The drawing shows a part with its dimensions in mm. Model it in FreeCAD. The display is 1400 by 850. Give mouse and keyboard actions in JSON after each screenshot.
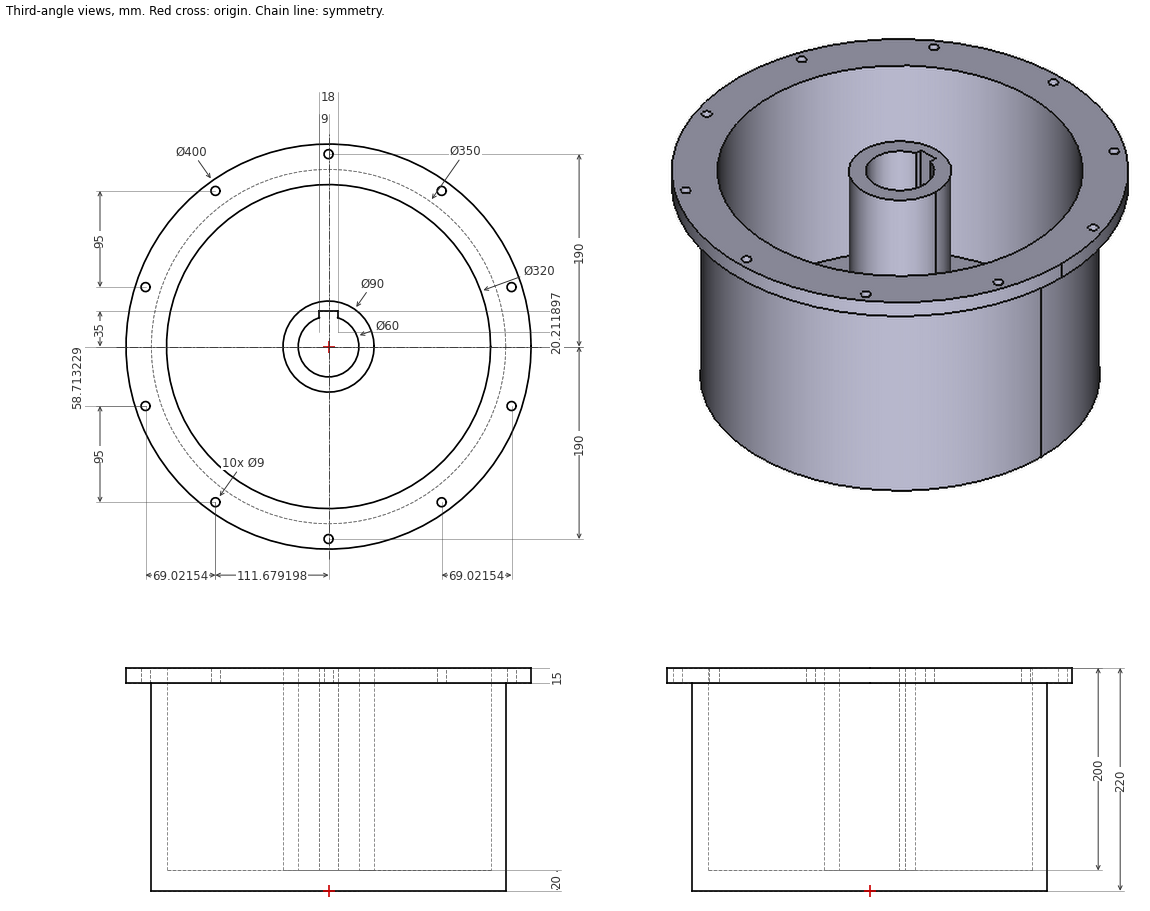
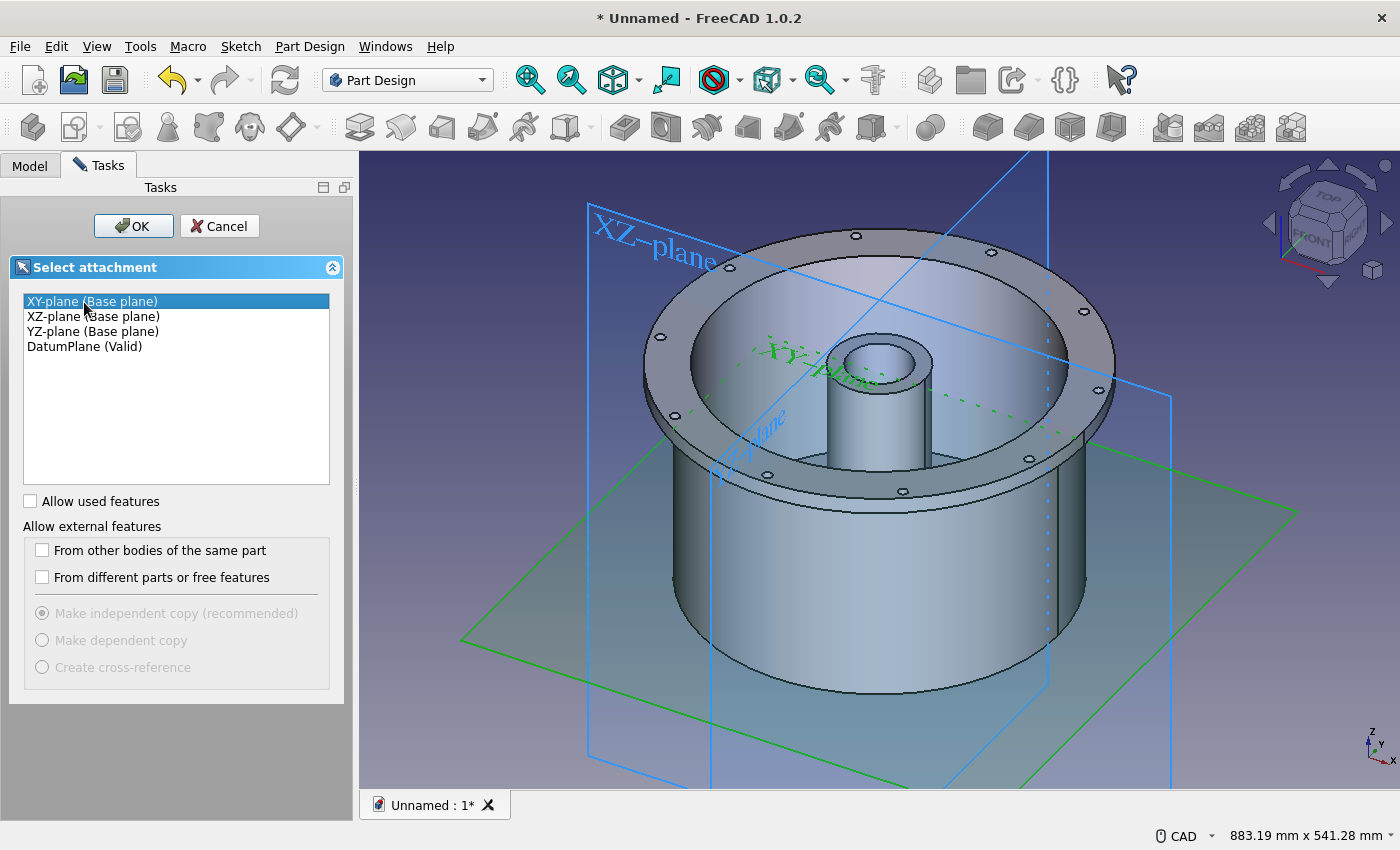
{"action": "left_click", "coordinate": [134, 226]}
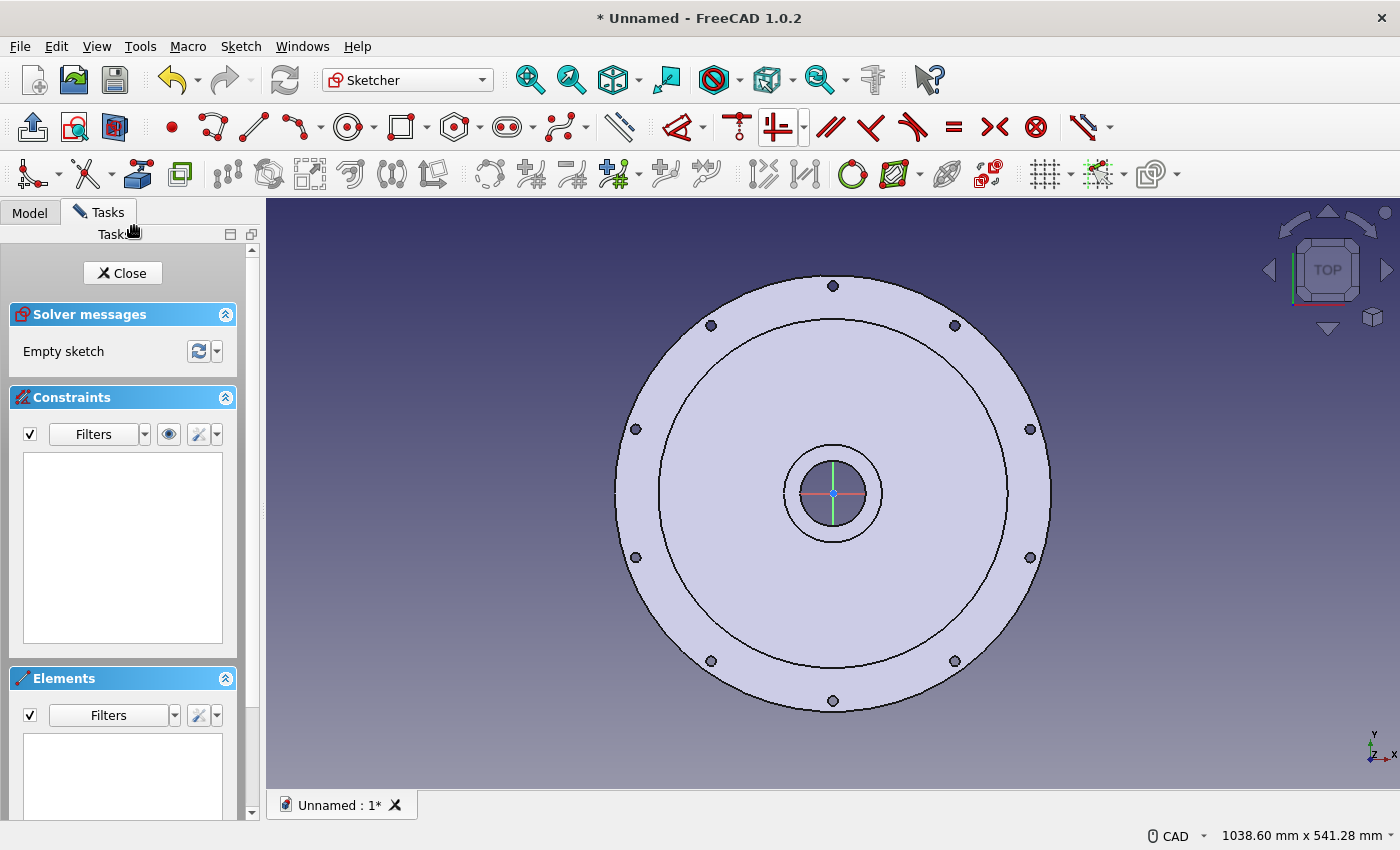
{"action": "left_click", "coordinate": [115, 128]}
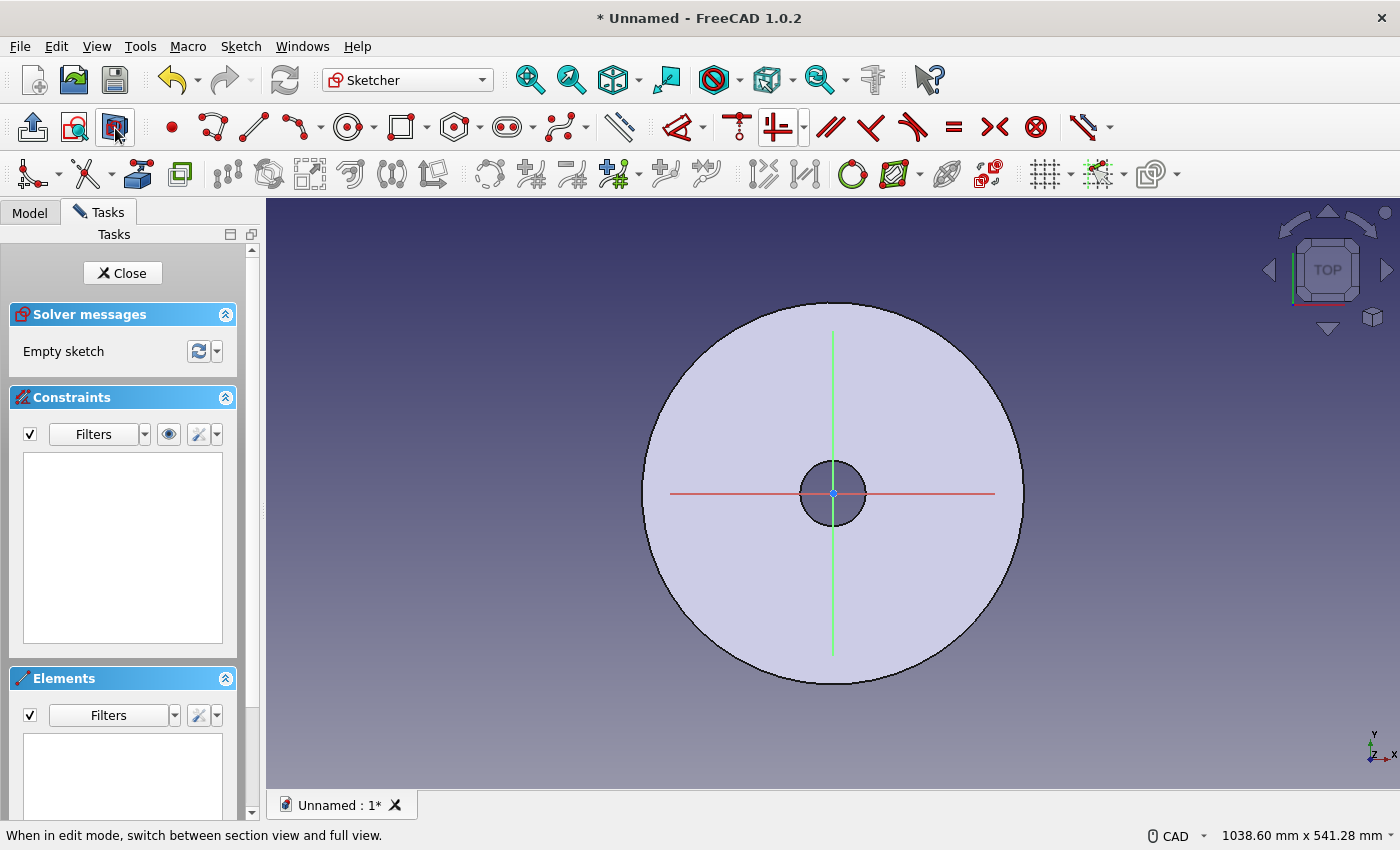
{"action": "scroll", "coordinate": [847, 494], "scroll_direction": "up", "scroll_amount": 9}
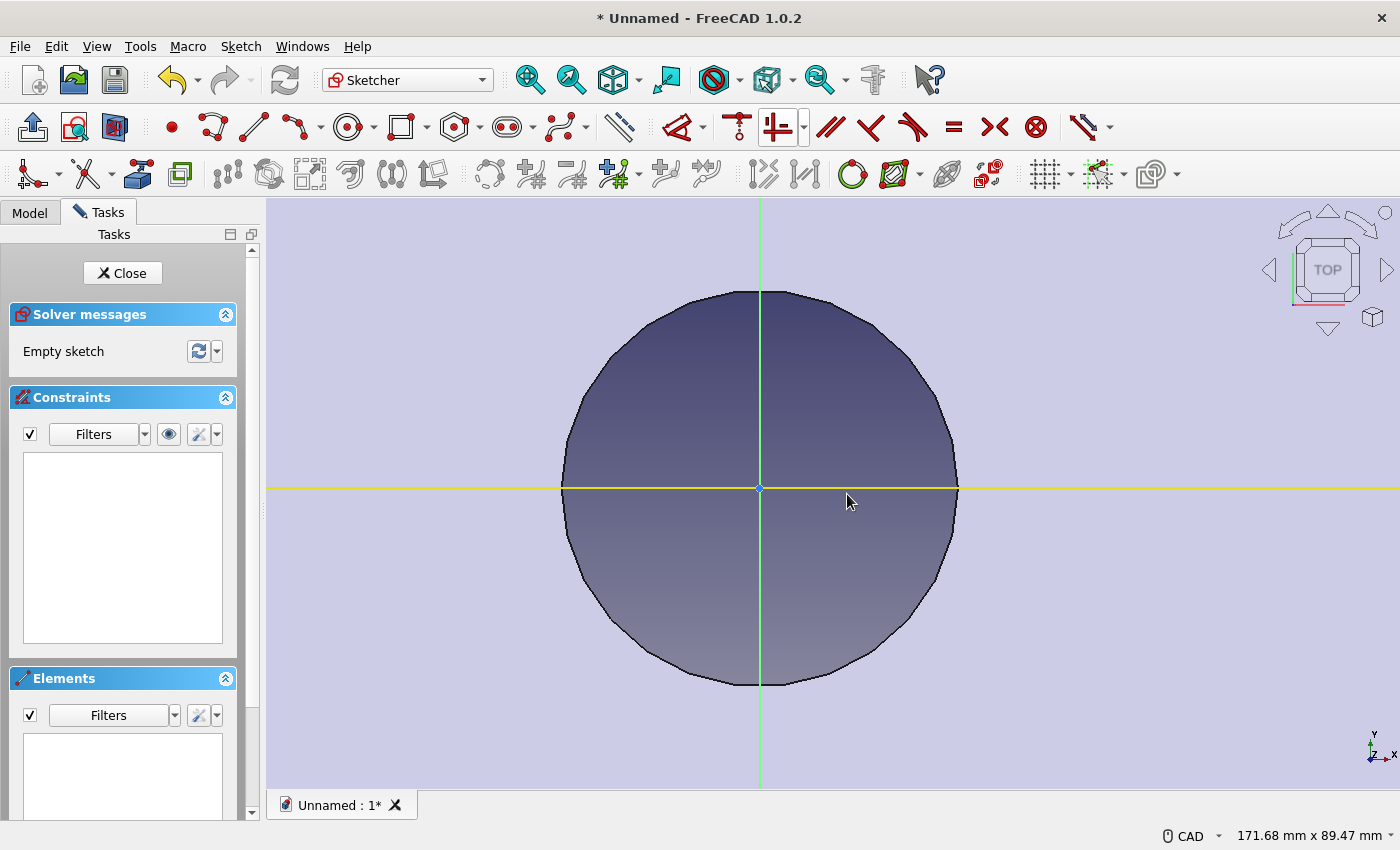
{"action": "left_click", "coordinate": [348, 128]}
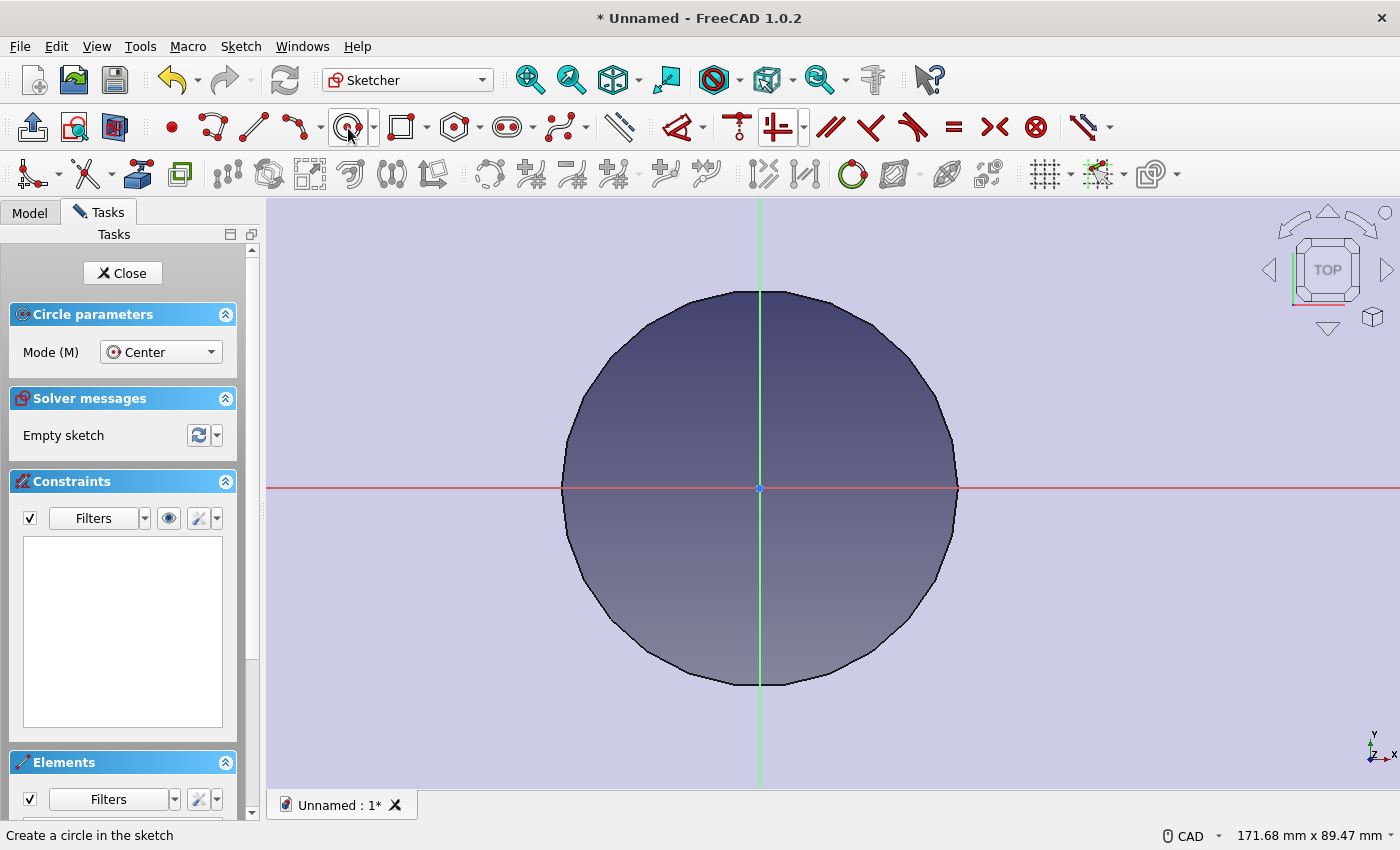
{"action": "left_click", "coordinate": [760, 488]}
{"action": "mouse_move", "coordinate": [900, 348]}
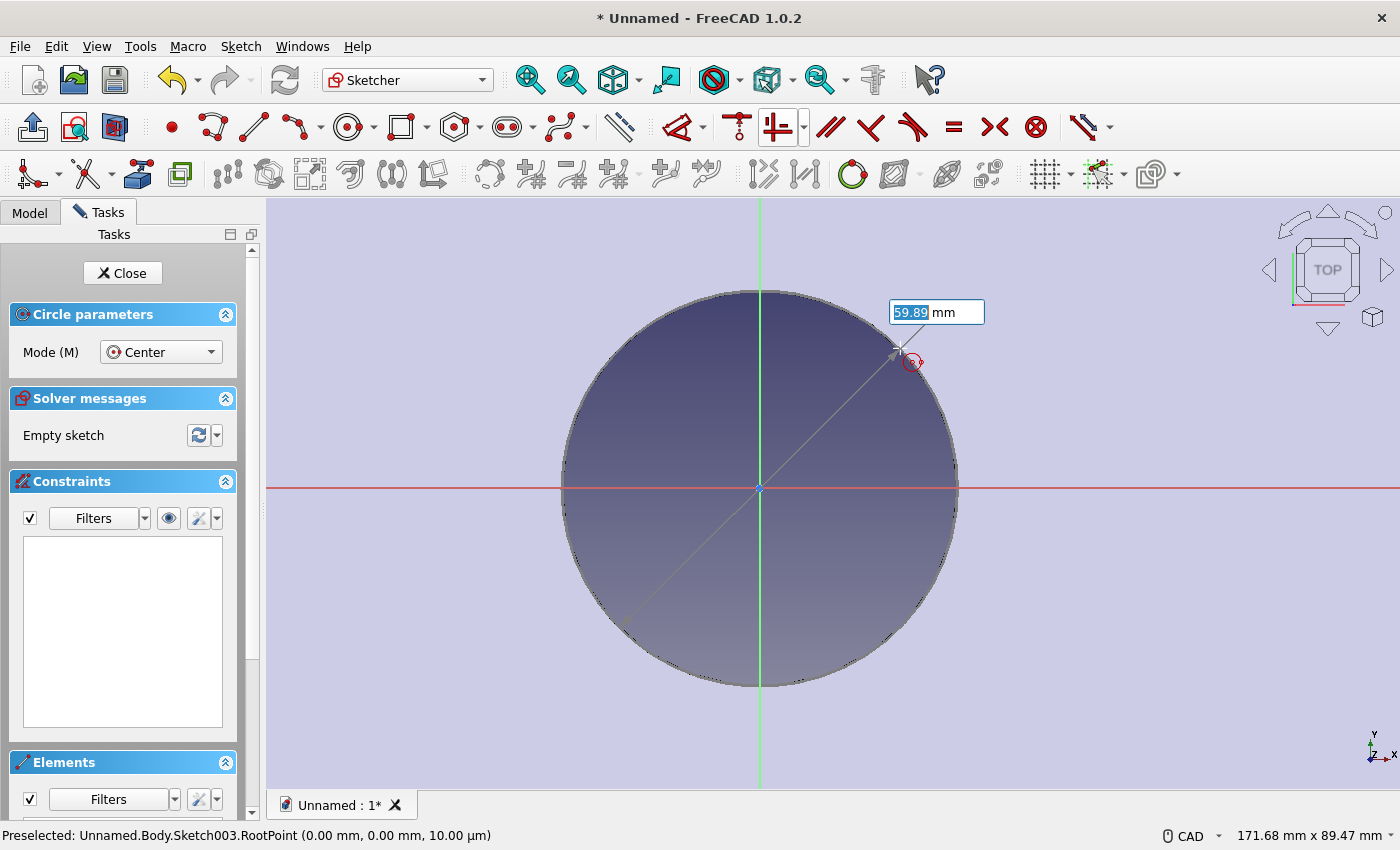
{"action": "type", "text": "60"}
{"action": "key", "text": "Return"}
{"action": "key", "text": "Escape"}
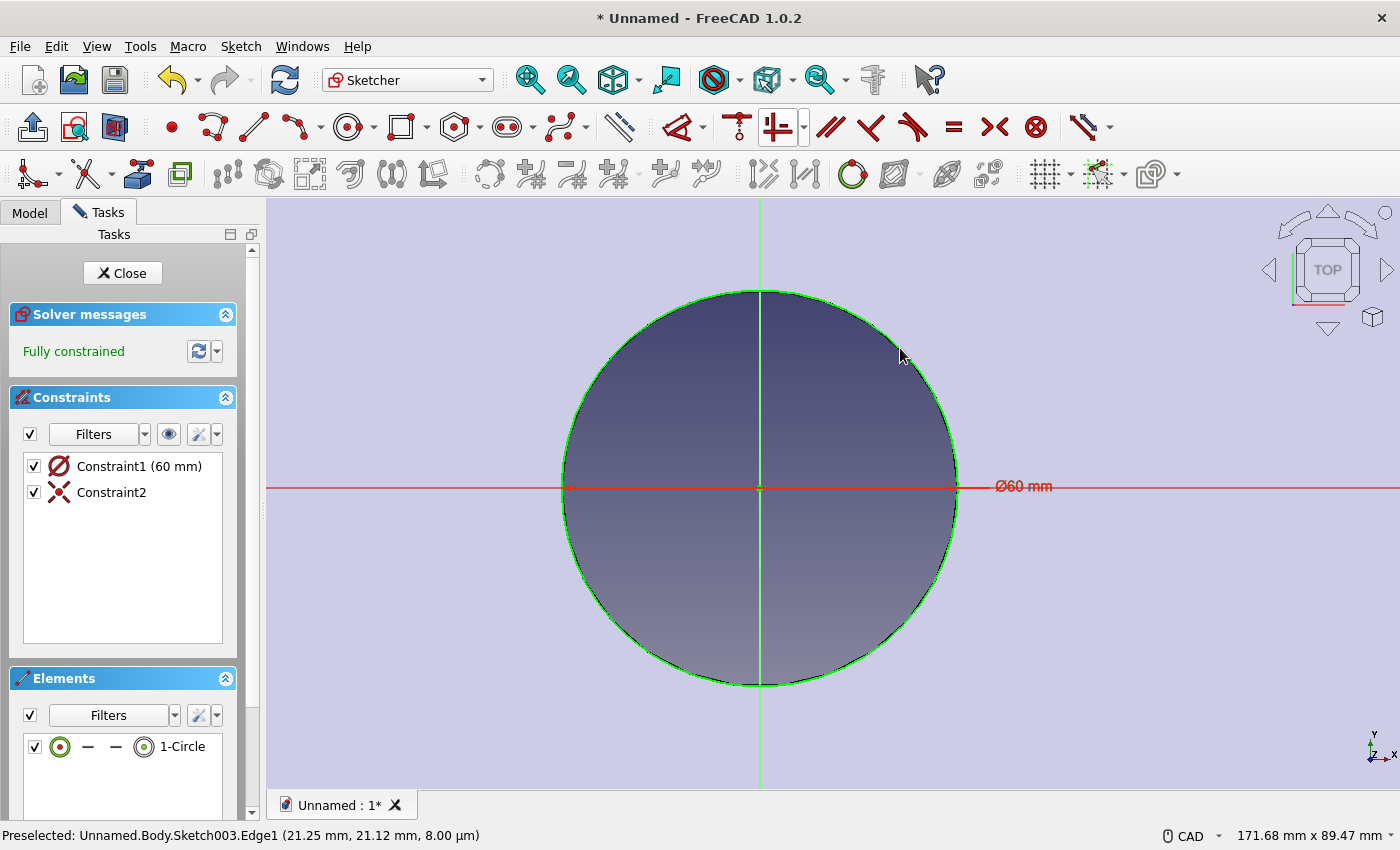
{"action": "left_click", "coordinate": [123, 273]}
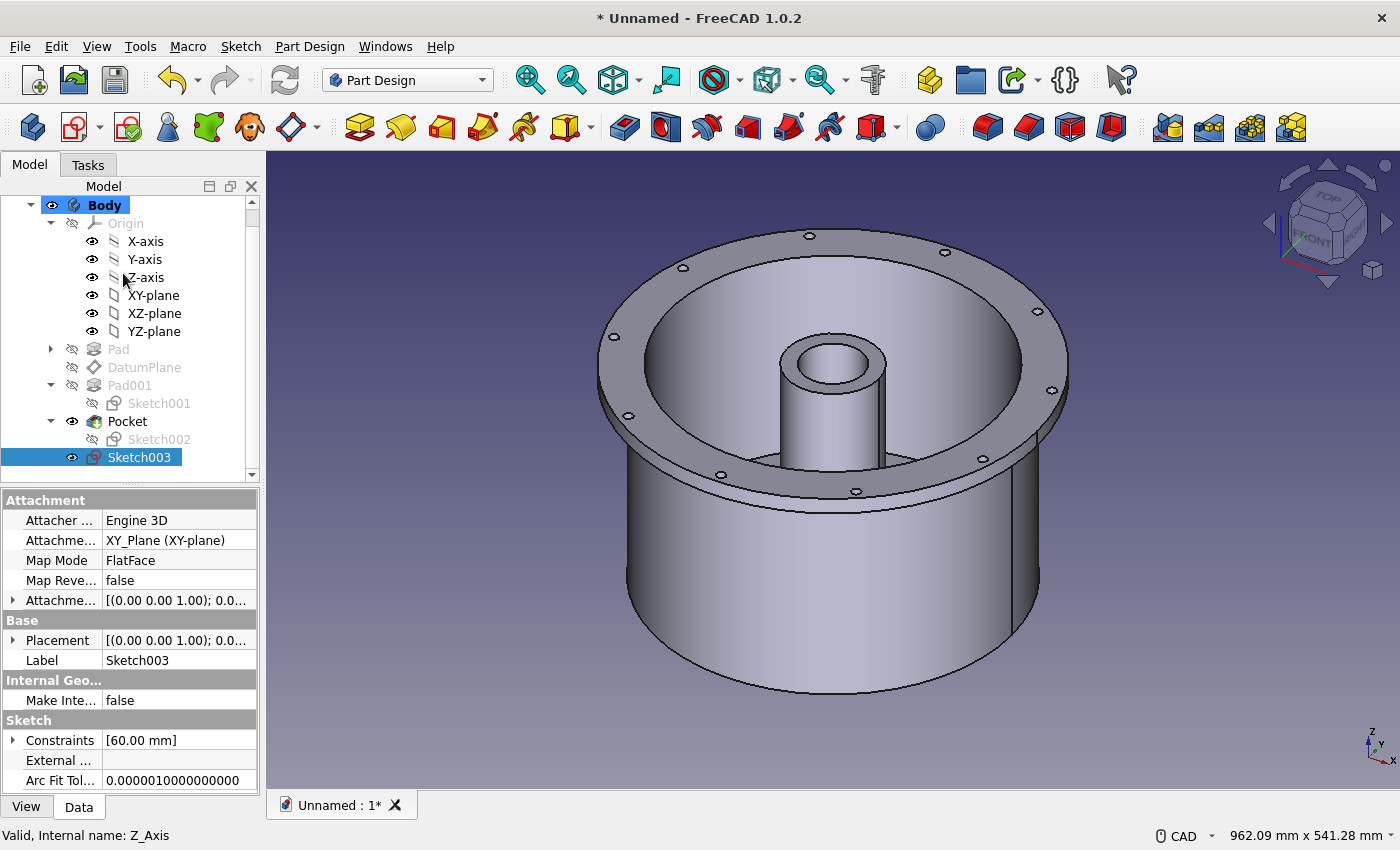
{"action": "left_click", "coordinate": [360, 128]}